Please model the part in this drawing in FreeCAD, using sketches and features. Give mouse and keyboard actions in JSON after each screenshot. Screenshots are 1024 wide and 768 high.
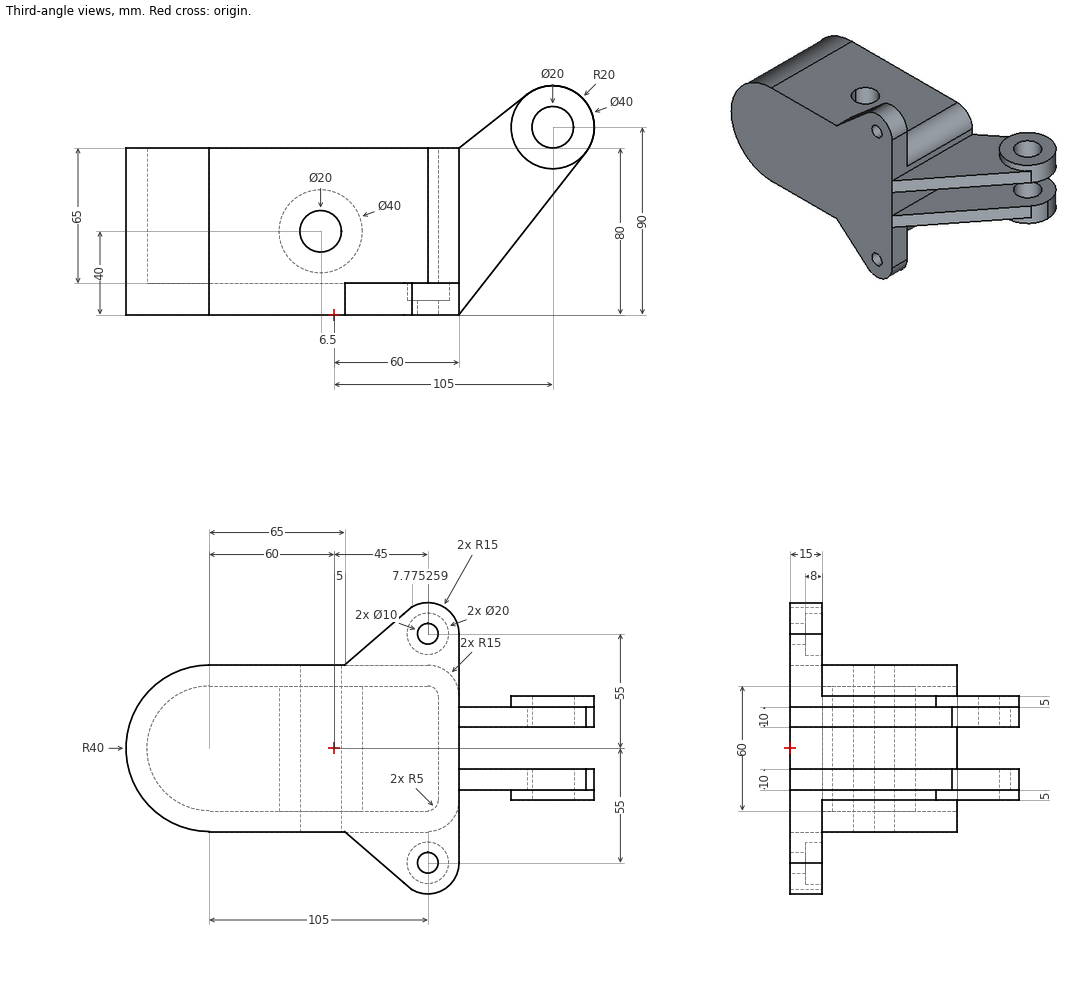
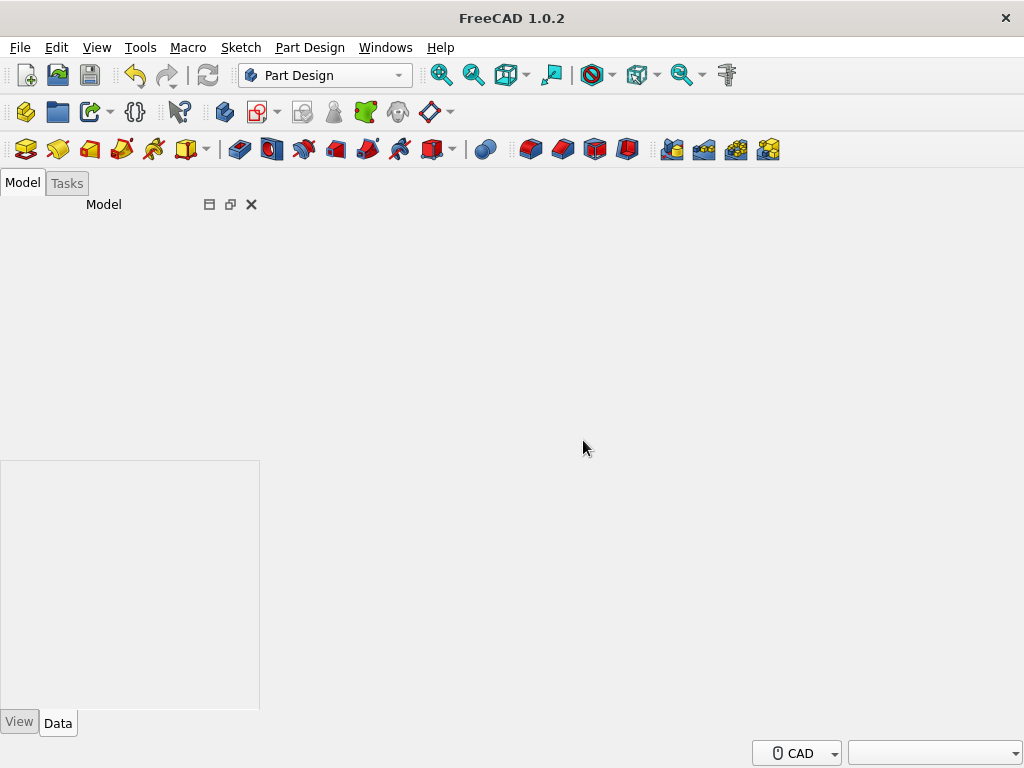
{"action": "left_click", "coordinate": [26, 76]}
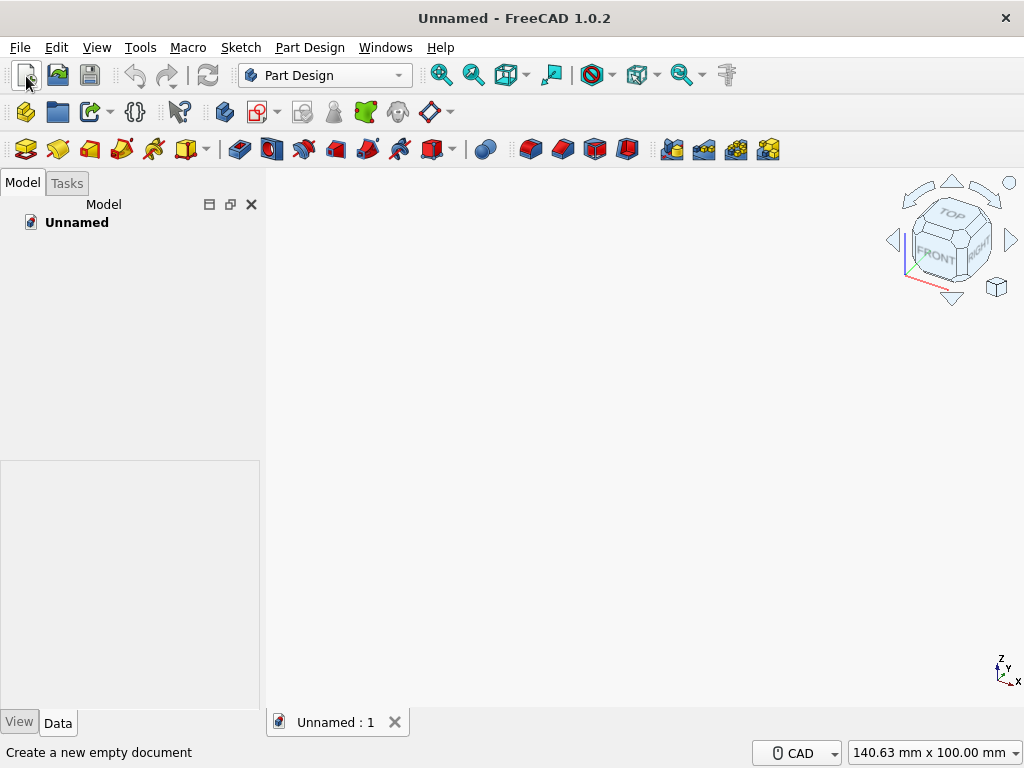
{"action": "left_click", "coordinate": [258, 112]}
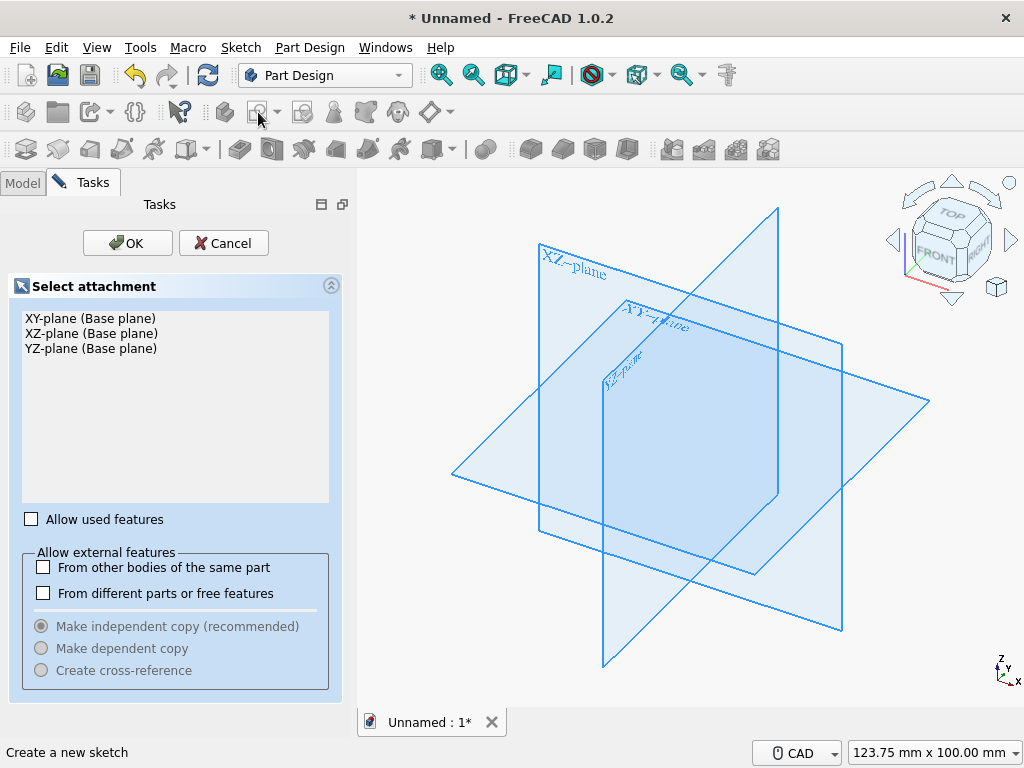
{"action": "left_click", "coordinate": [82, 334]}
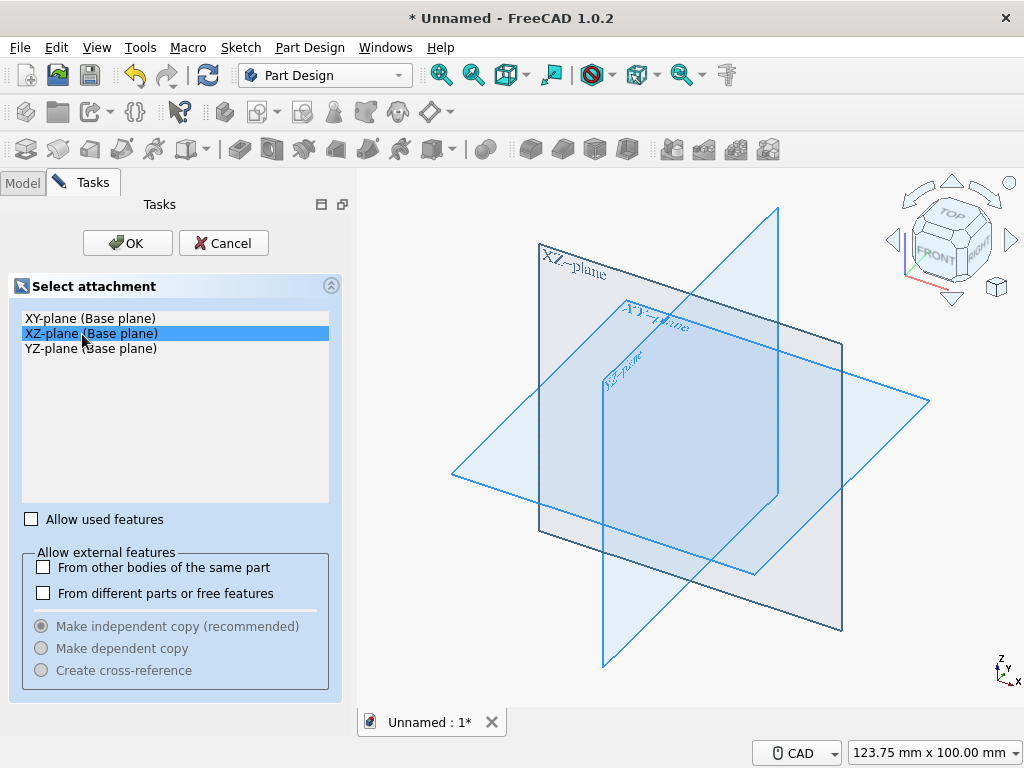
{"action": "left_click", "coordinate": [128, 243]}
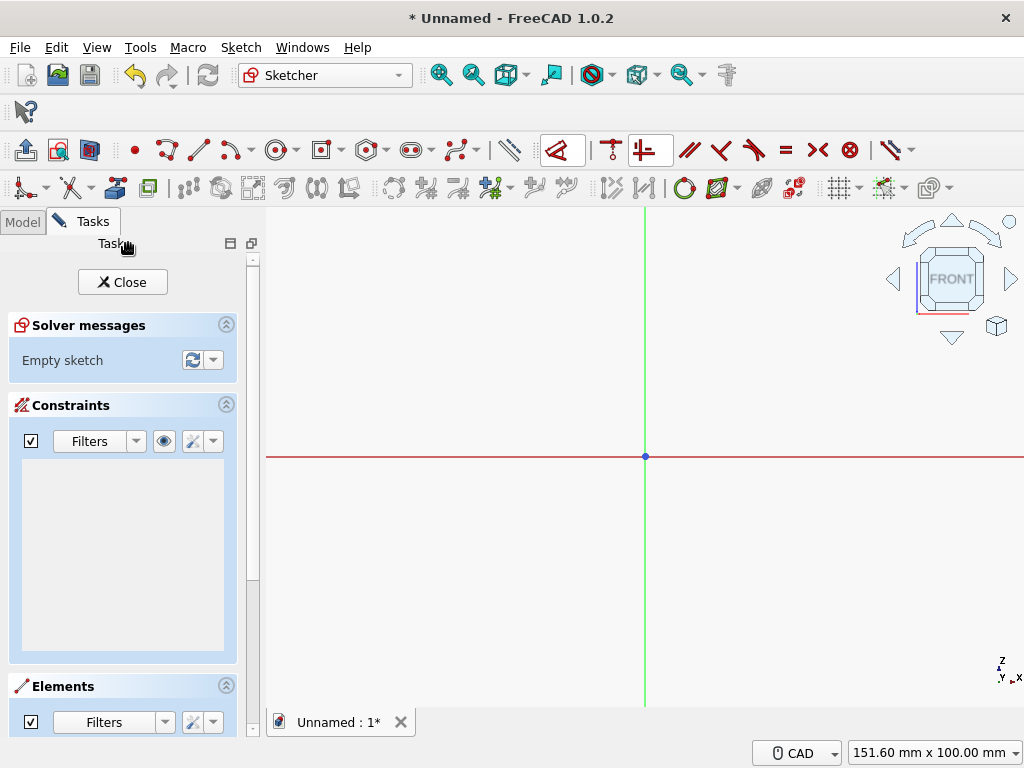
{"action": "scroll", "coordinate": [602, 457], "scroll_direction": "down", "scroll_amount": 4}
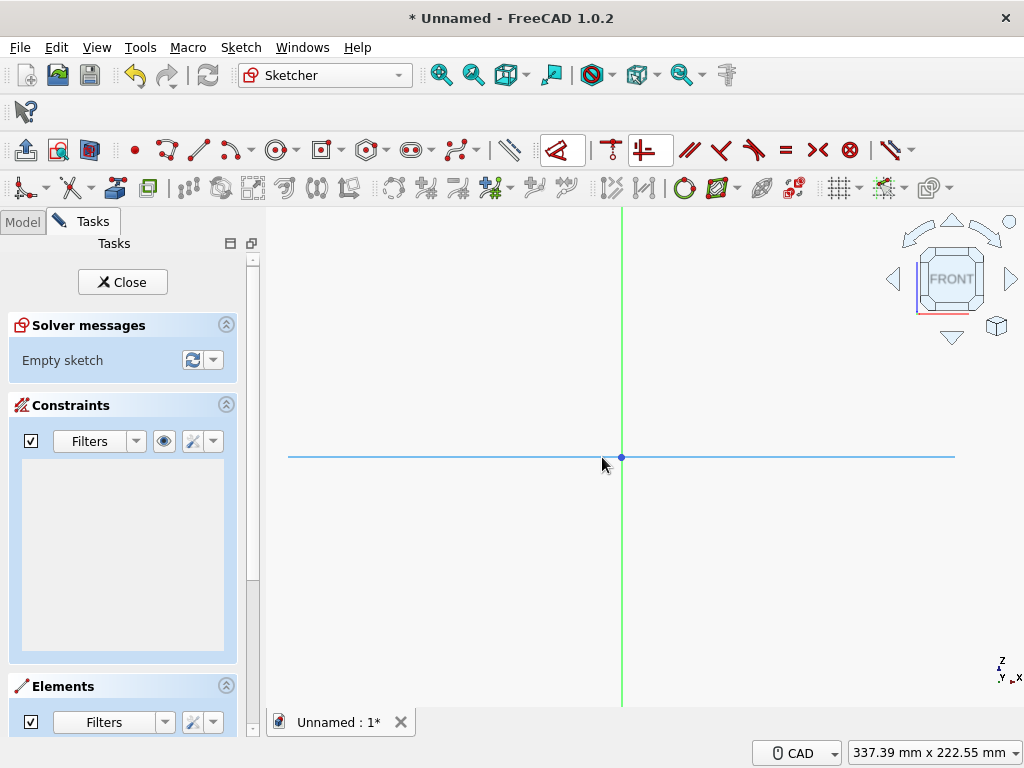
{"action": "left_click", "coordinate": [168, 150]}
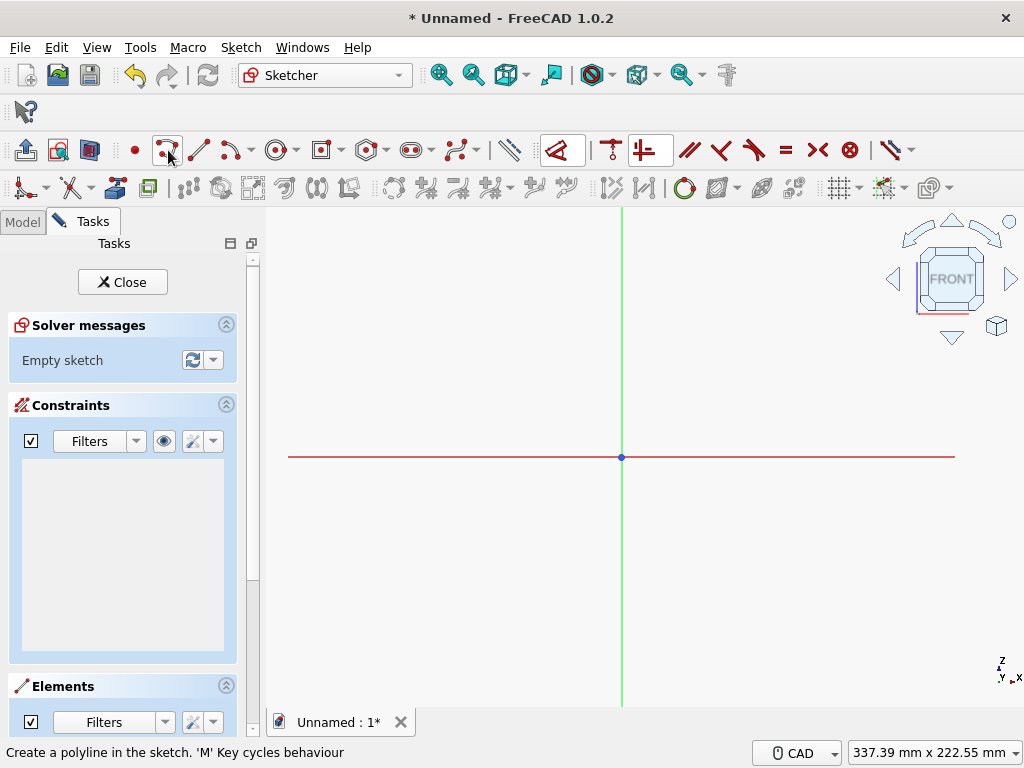
{"action": "left_click", "coordinate": [487, 367]}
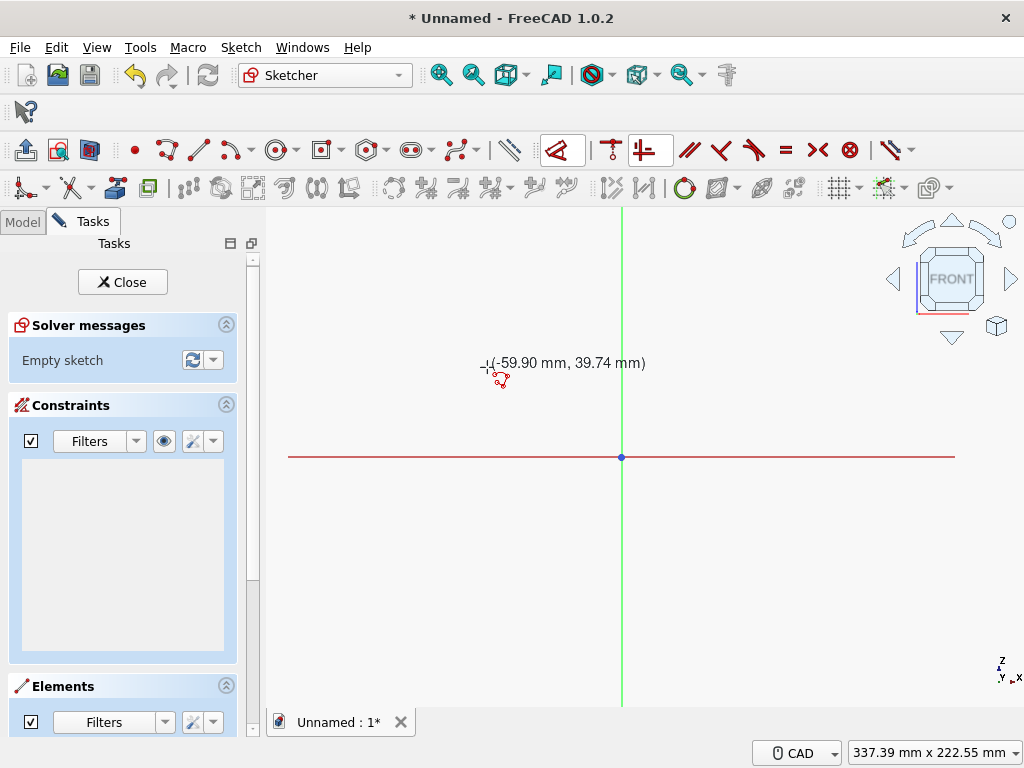
{"action": "scroll", "coordinate": [633, 367], "scroll_direction": "up", "scroll_amount": 2}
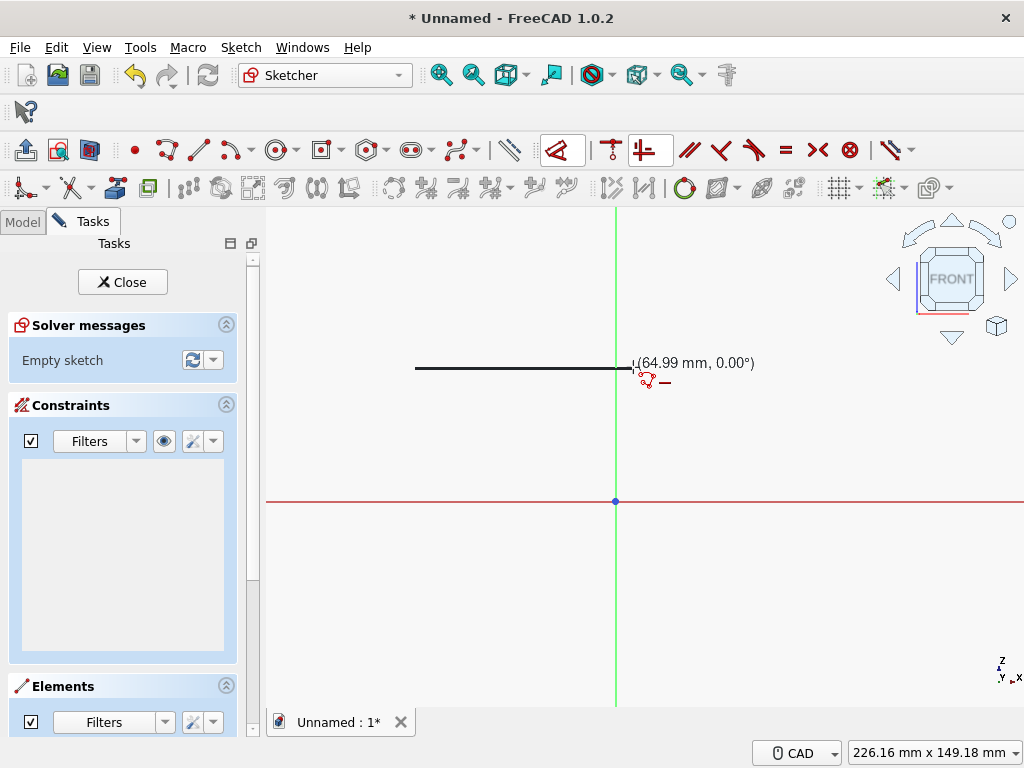
{"action": "left_click", "coordinate": [632, 367]}
{"action": "left_click", "coordinate": [740, 274]}
{"action": "right_click", "coordinate": [740, 274]}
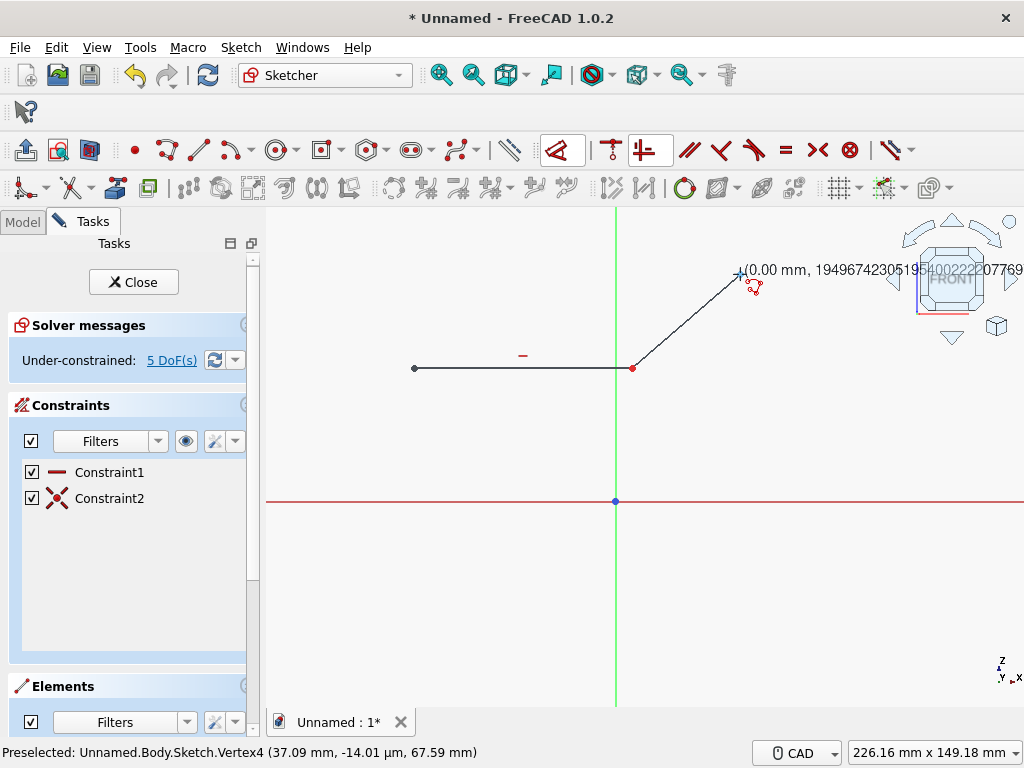
{"action": "left_click", "coordinate": [200, 150]}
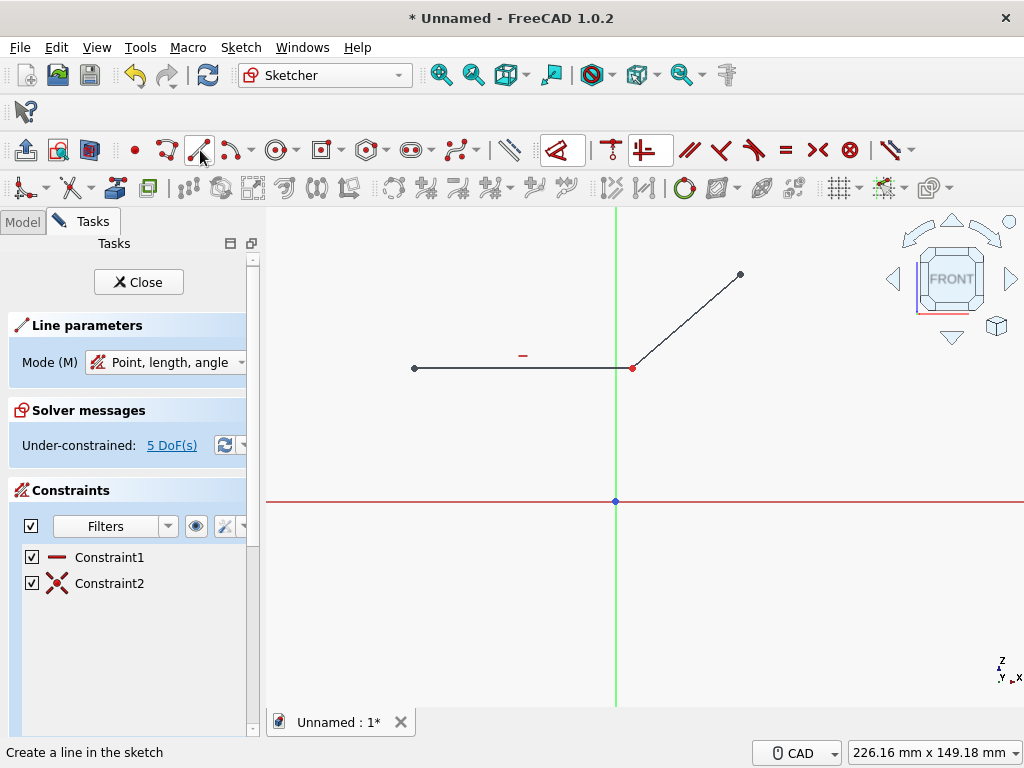
{"action": "left_click", "coordinate": [817, 317]}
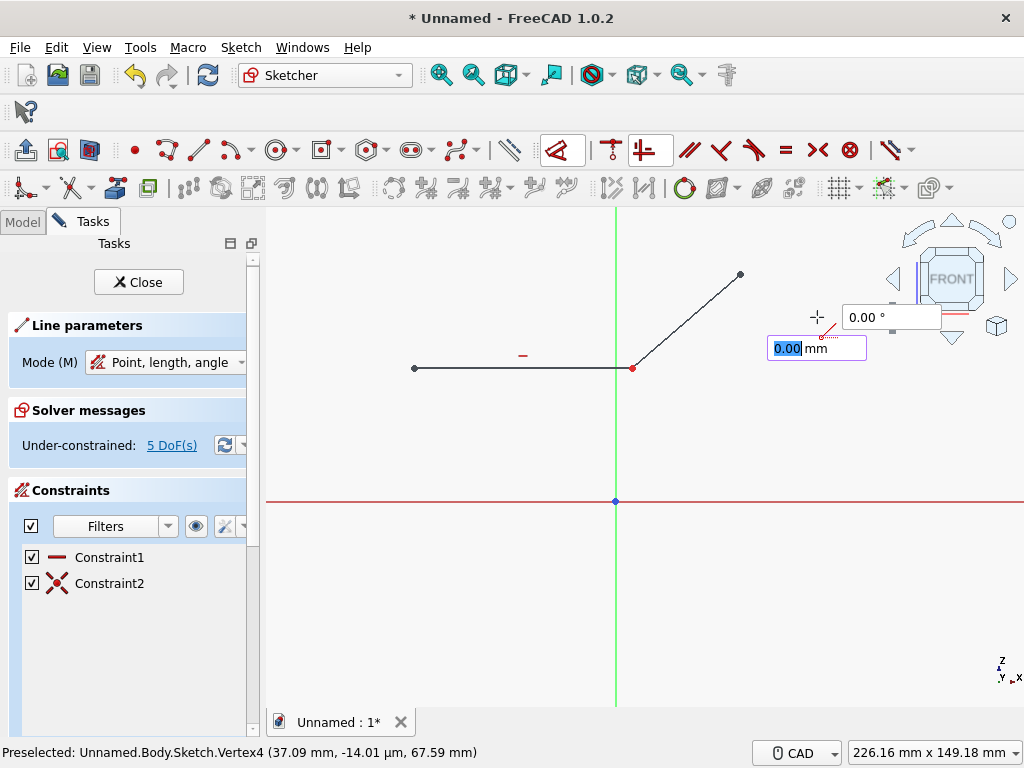
{"action": "scroll", "coordinate": [633, 366], "scroll_direction": "down", "scroll_amount": 2}